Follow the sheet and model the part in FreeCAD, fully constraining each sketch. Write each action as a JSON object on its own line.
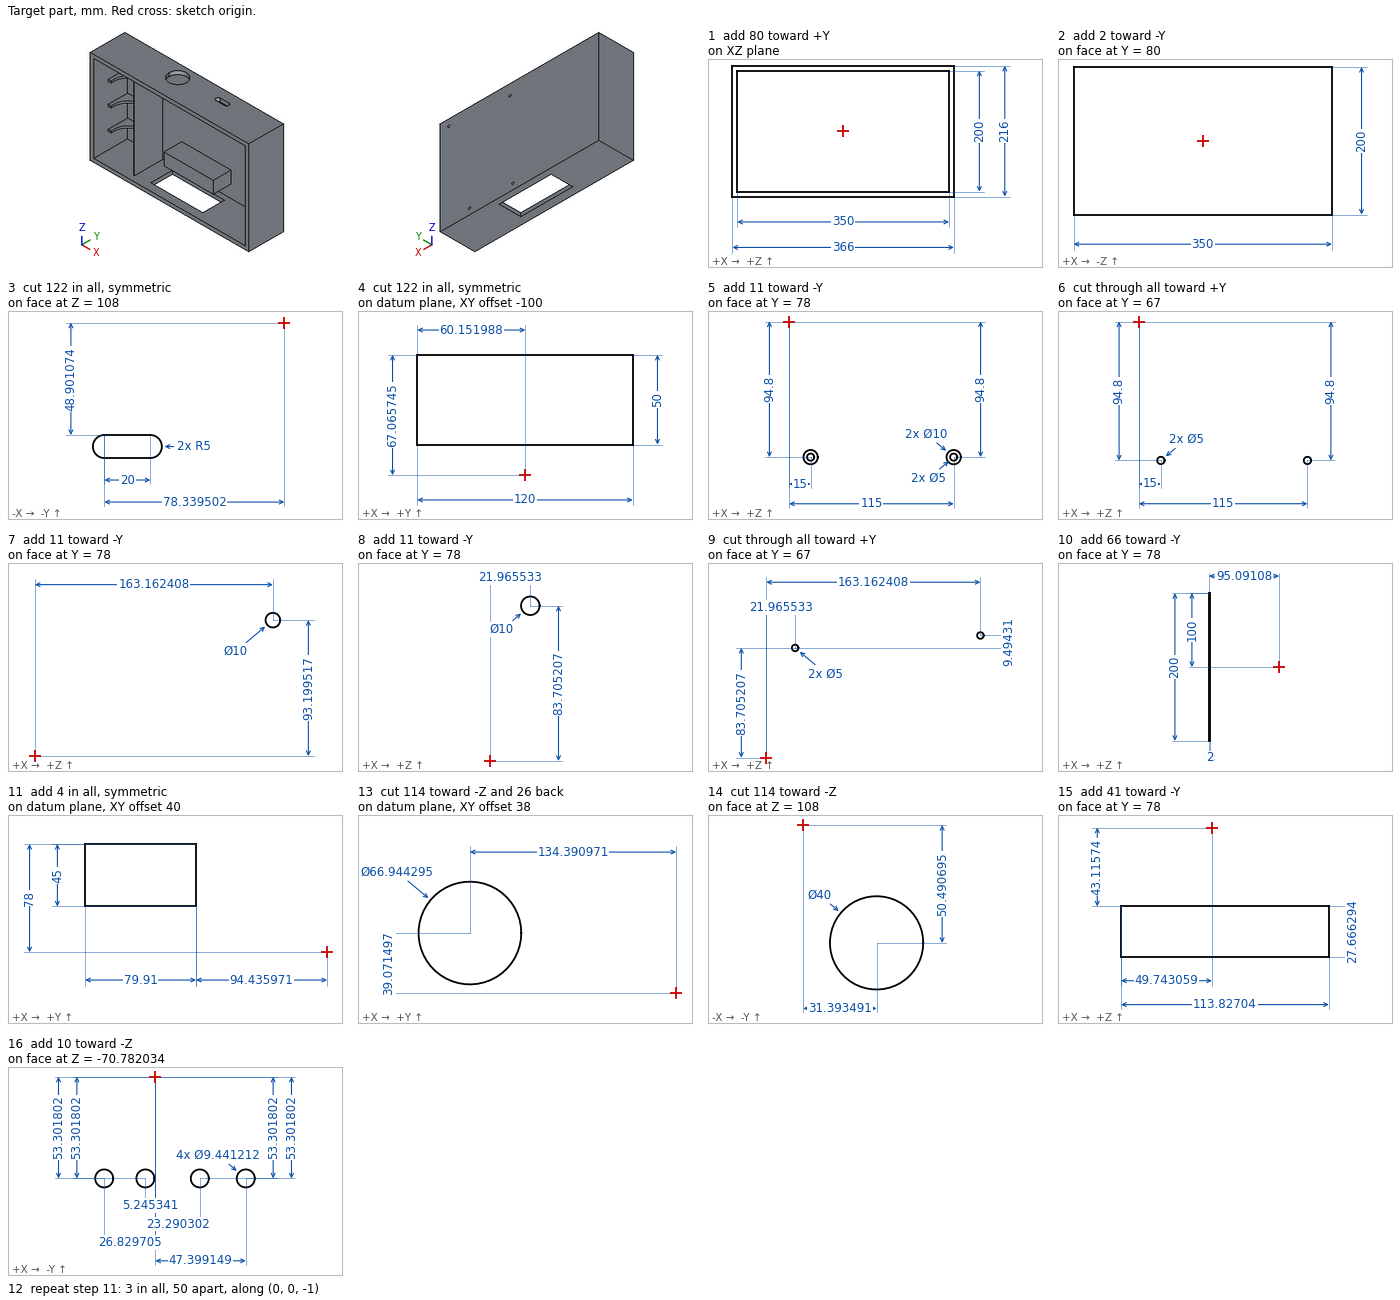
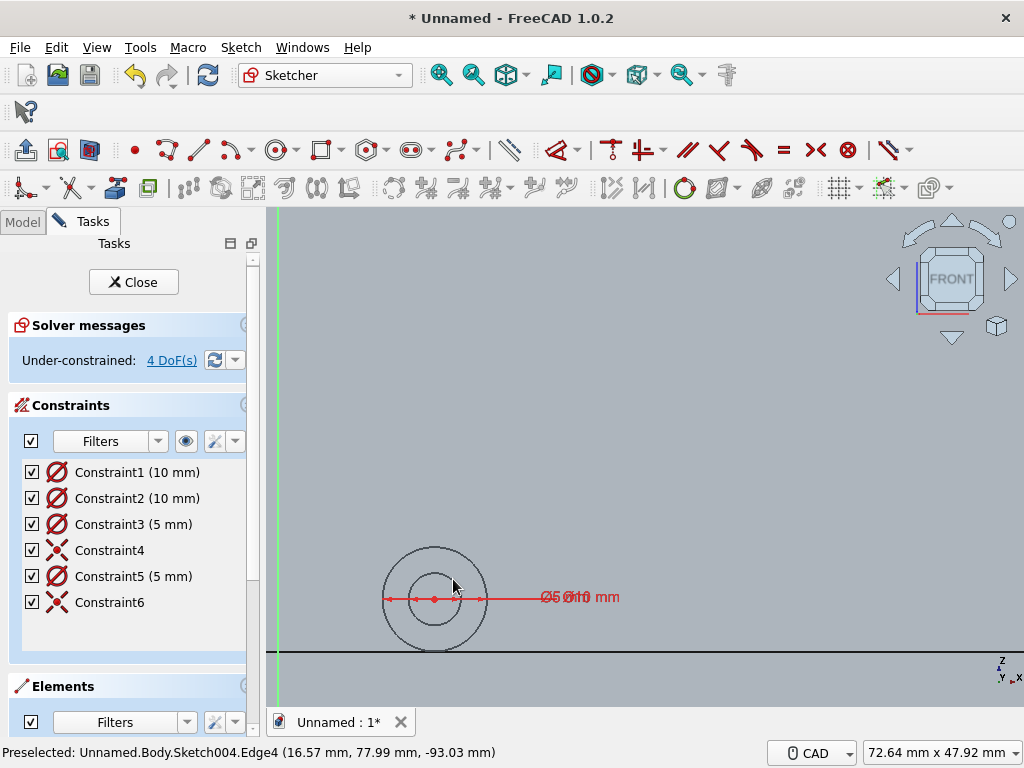
{"action": "key", "text": "d"}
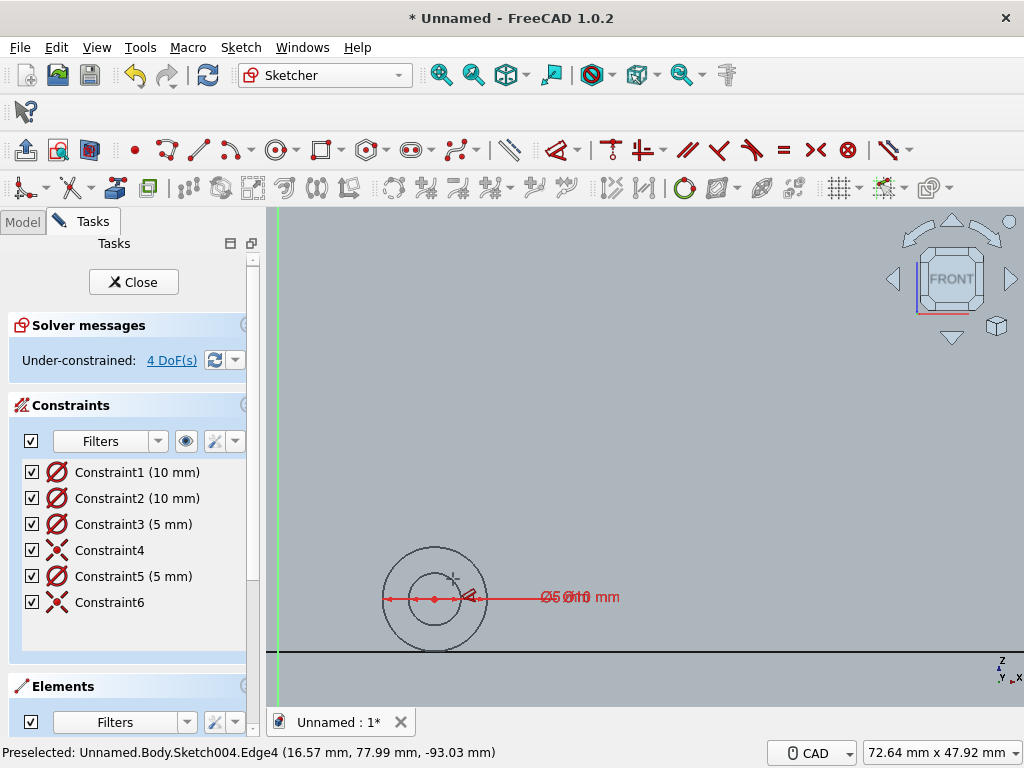
{"action": "left_click", "coordinate": [435, 599]}
{"action": "left_click", "coordinate": [364, 633]}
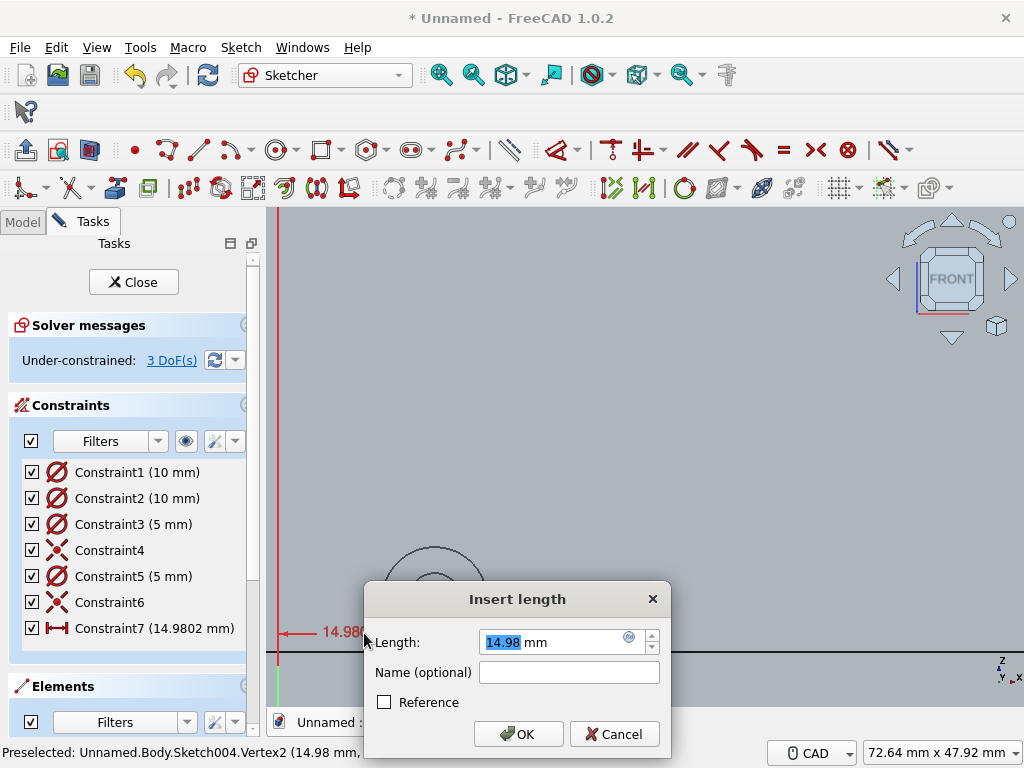
{"action": "type", "text": "15"}
{"action": "key", "text": "Return"}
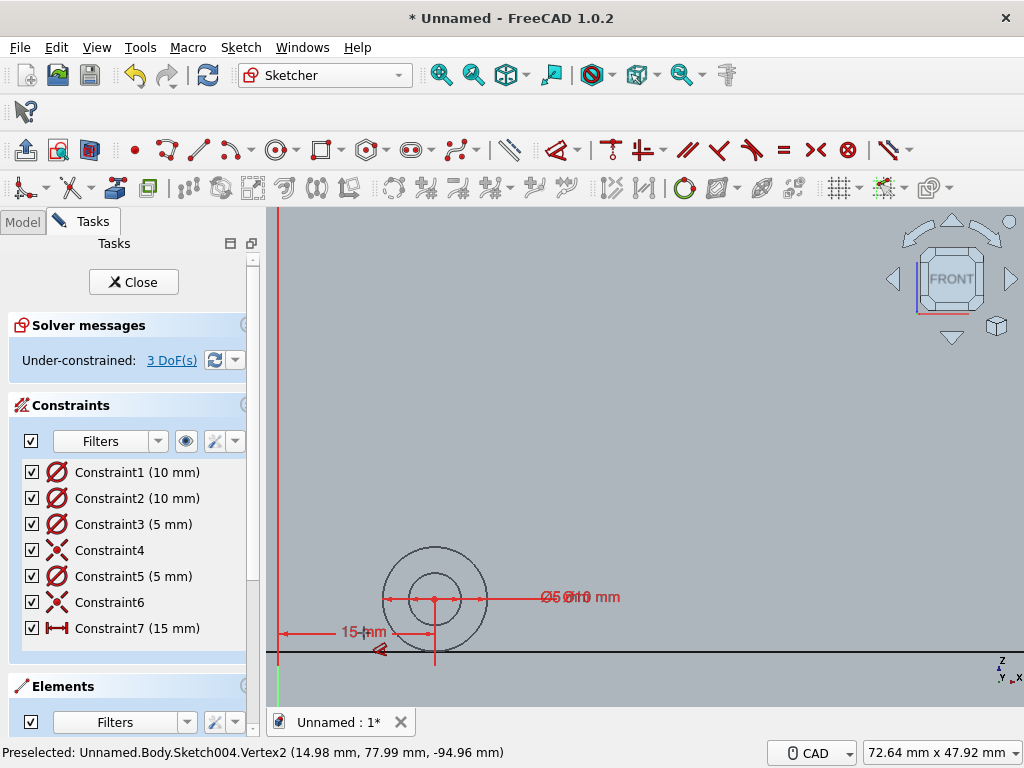
{"action": "scroll", "coordinate": [435, 598], "scroll_direction": "down", "scroll_amount": 6}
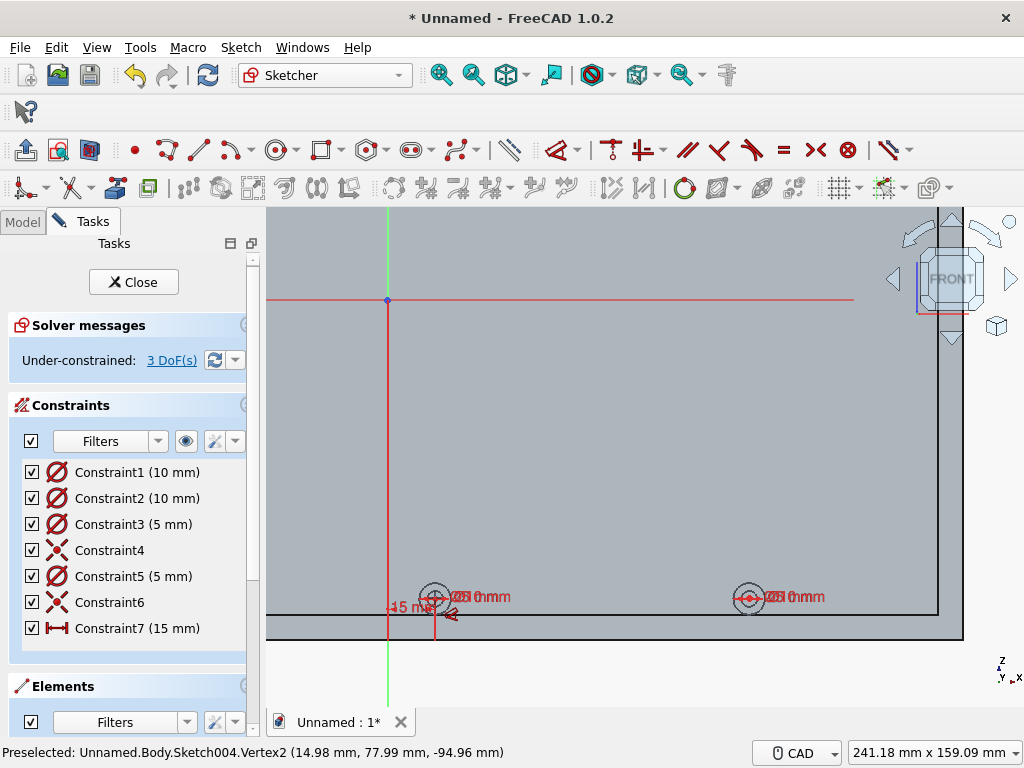
{"action": "left_click", "coordinate": [749, 599]}
{"action": "left_click", "coordinate": [569, 266]}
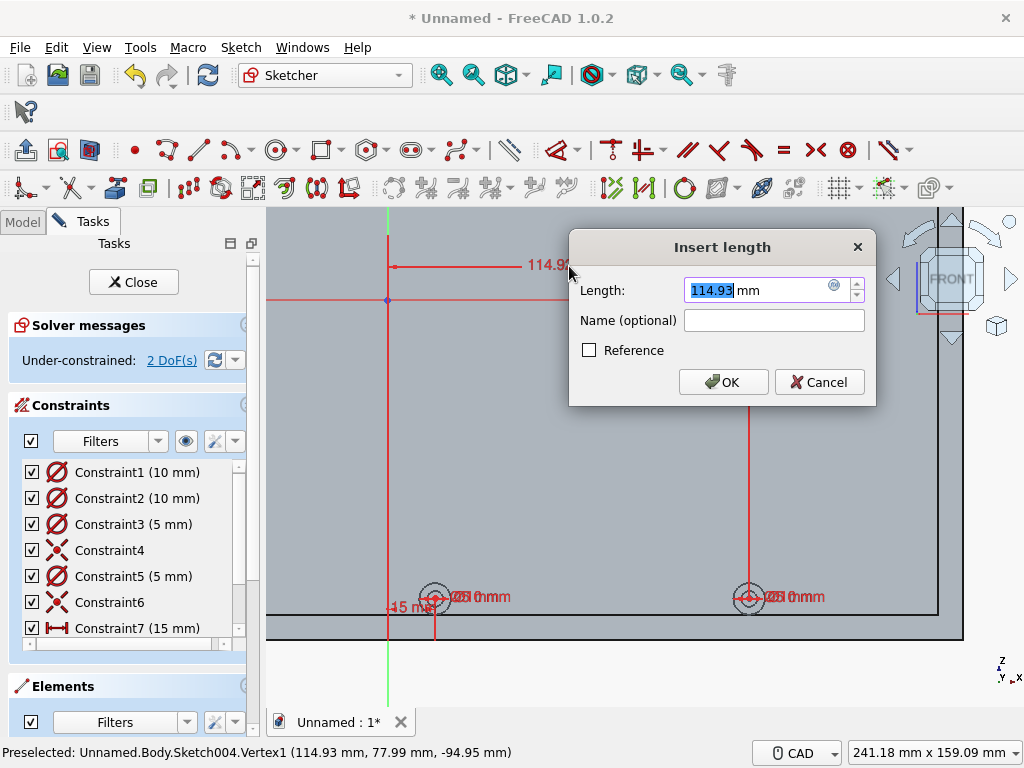
{"action": "type", "text": "115"}
{"action": "key", "text": "Return"}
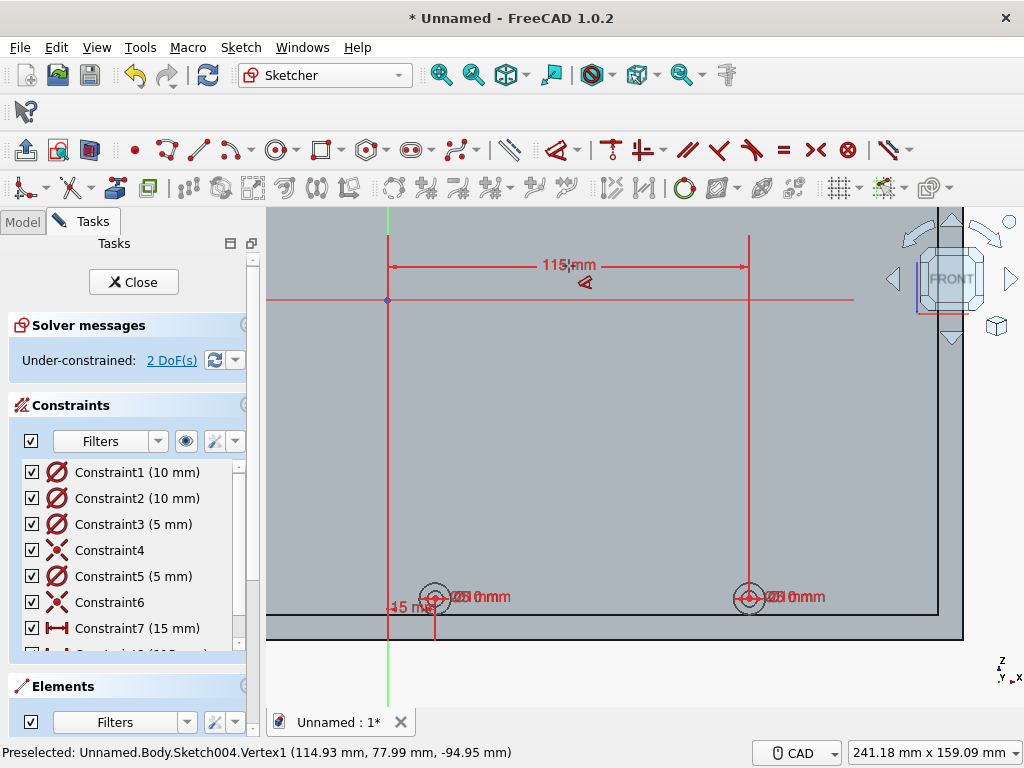
{"action": "left_click", "coordinate": [749, 599]}
{"action": "left_click", "coordinate": [354, 450]}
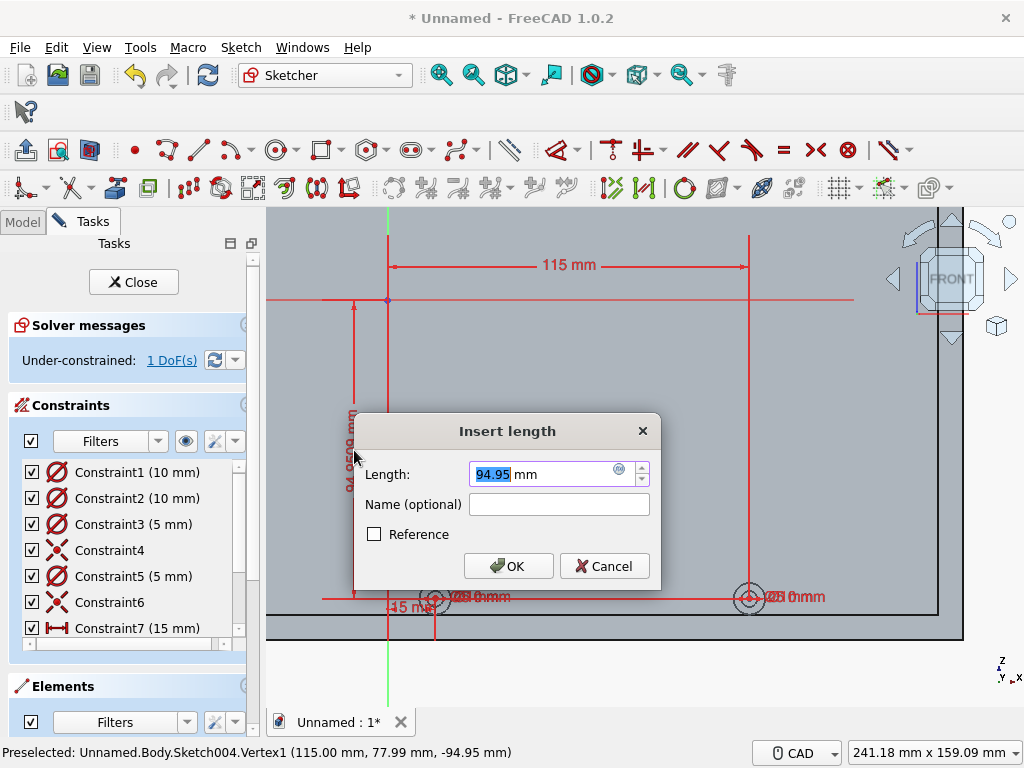
{"action": "type", "text": "94.8"}
{"action": "key", "text": "Return"}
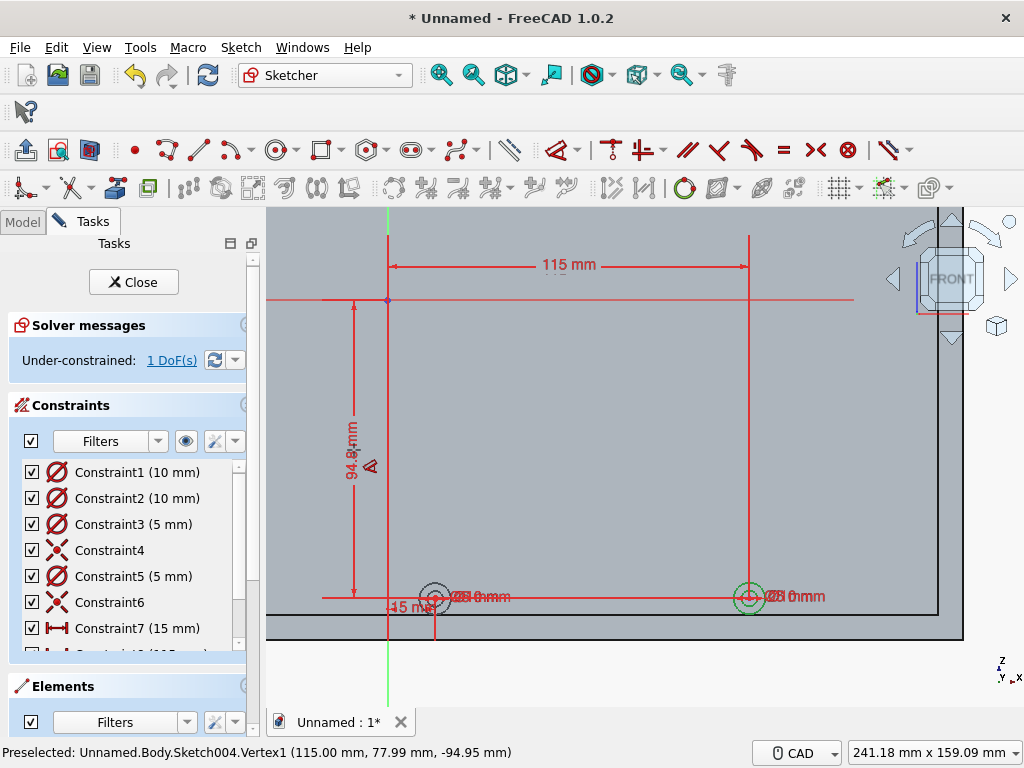
{"action": "left_click", "coordinate": [435, 599]}
{"action": "left_click", "coordinate": [354, 381]}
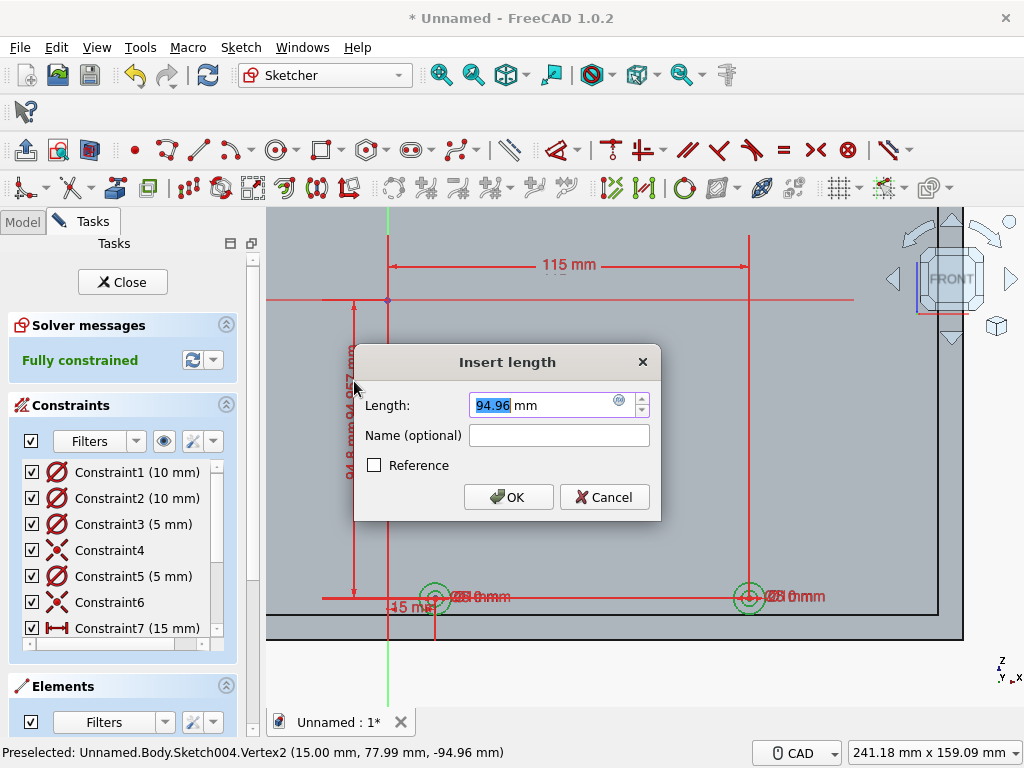
{"action": "type", "text": "94.8"}
{"action": "key", "text": "Return"}
{"action": "key", "text": "Escape"}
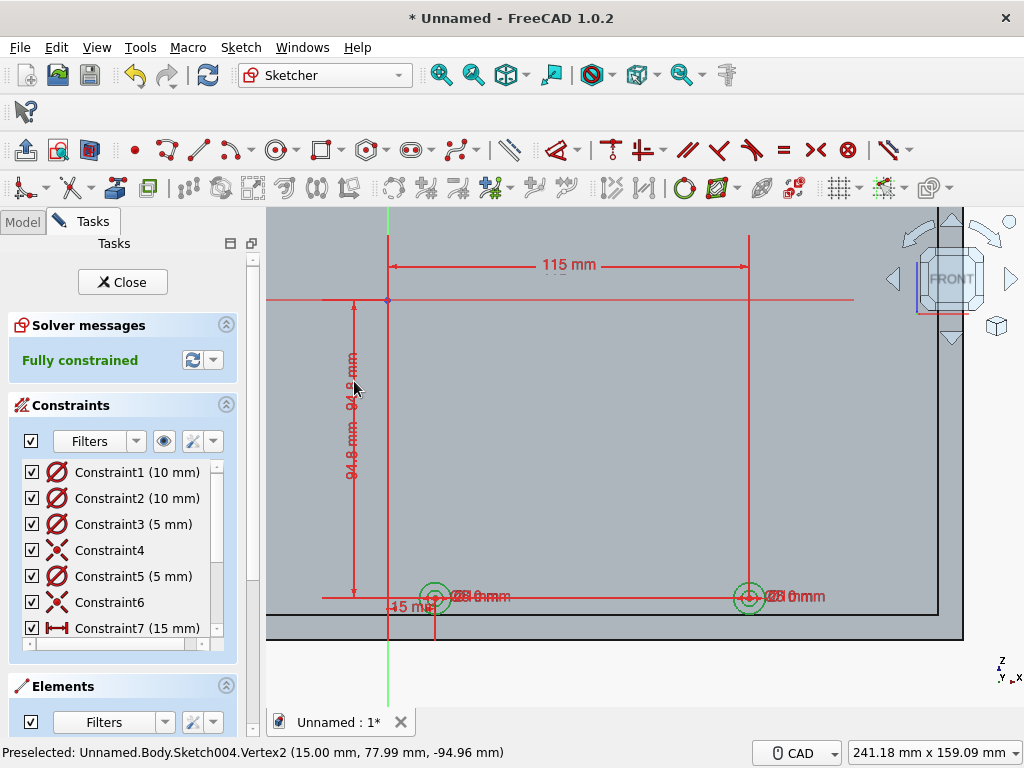
{"action": "left_click", "coordinate": [123, 282]}